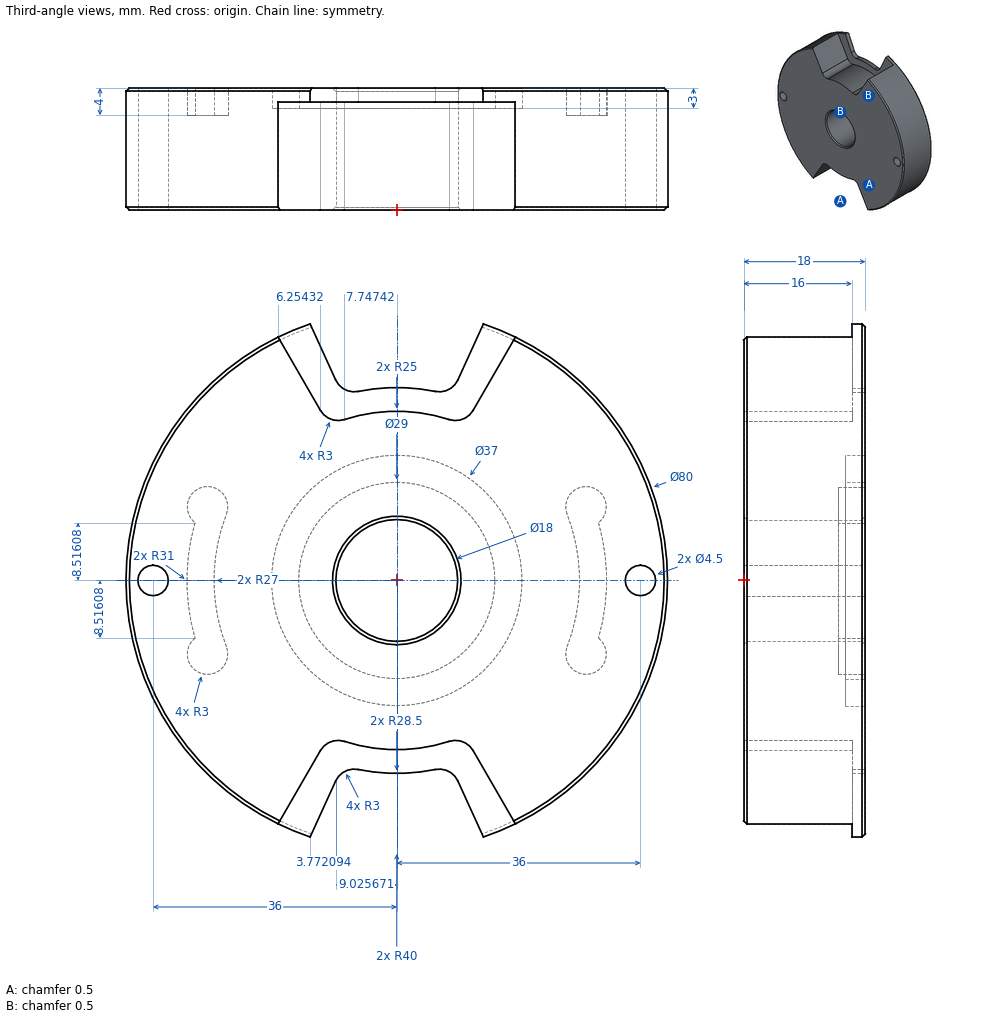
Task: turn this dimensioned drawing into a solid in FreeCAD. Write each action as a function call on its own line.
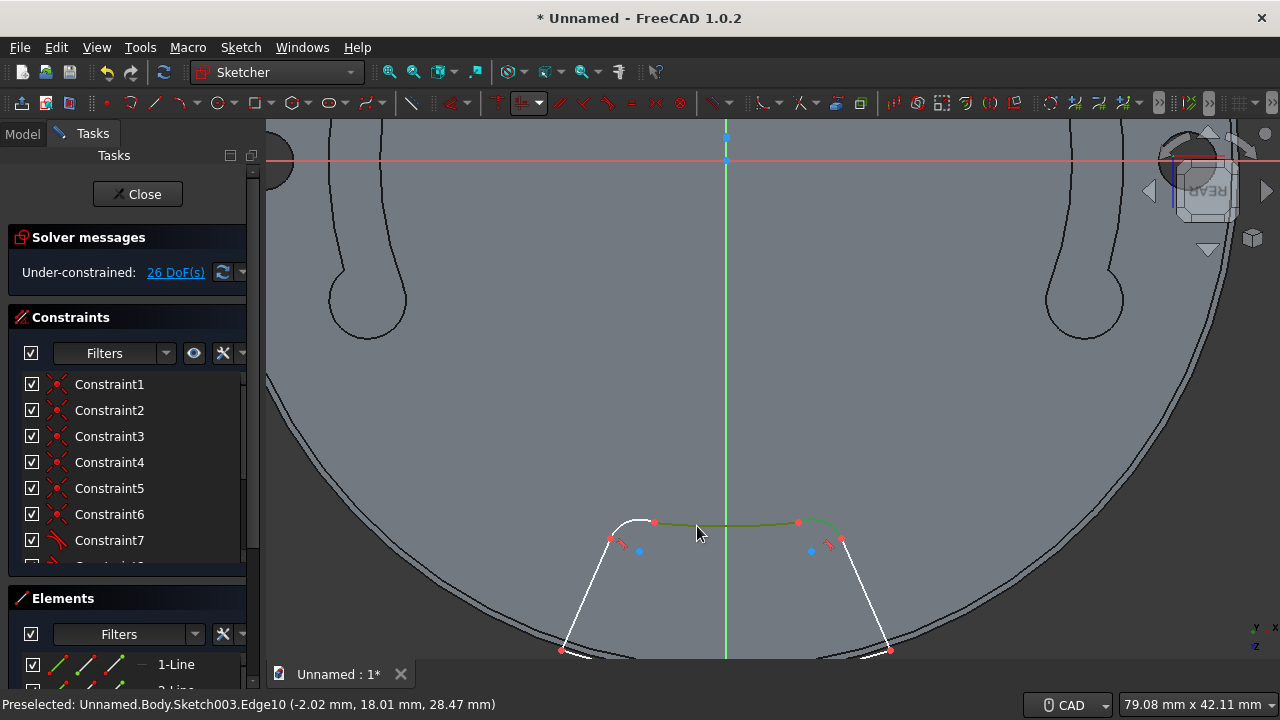
click(608, 104)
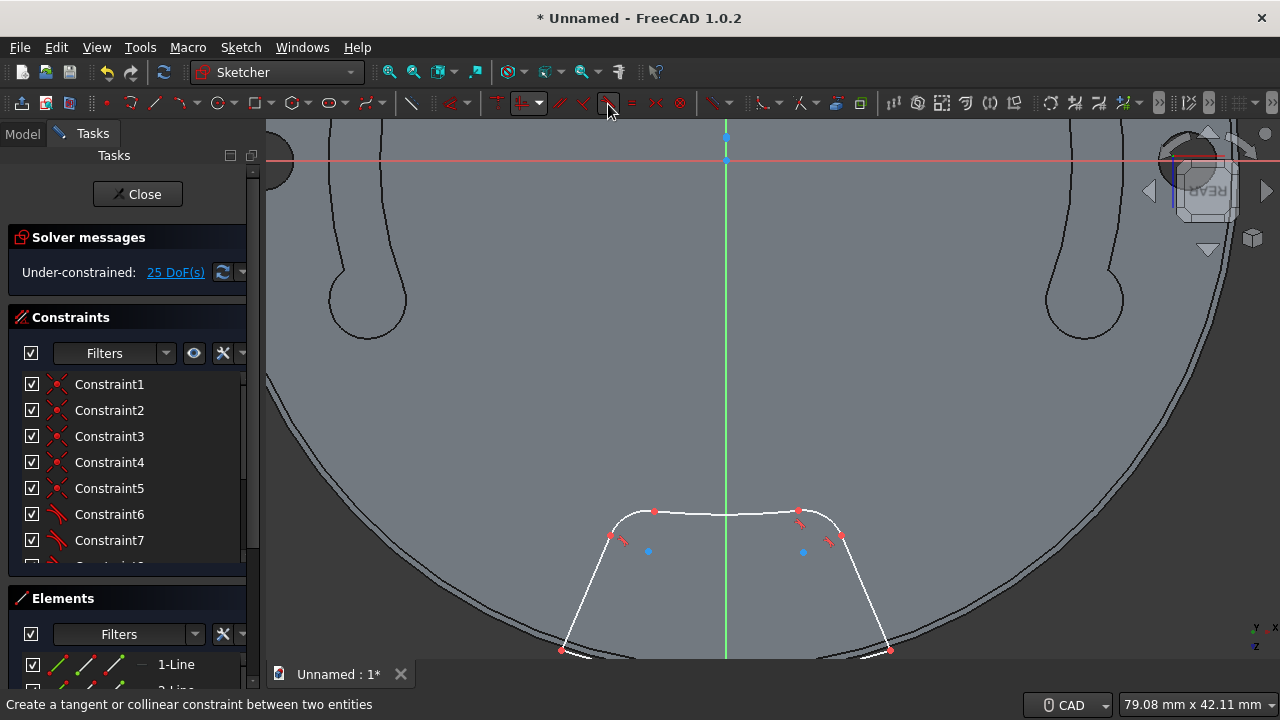
click(697, 514)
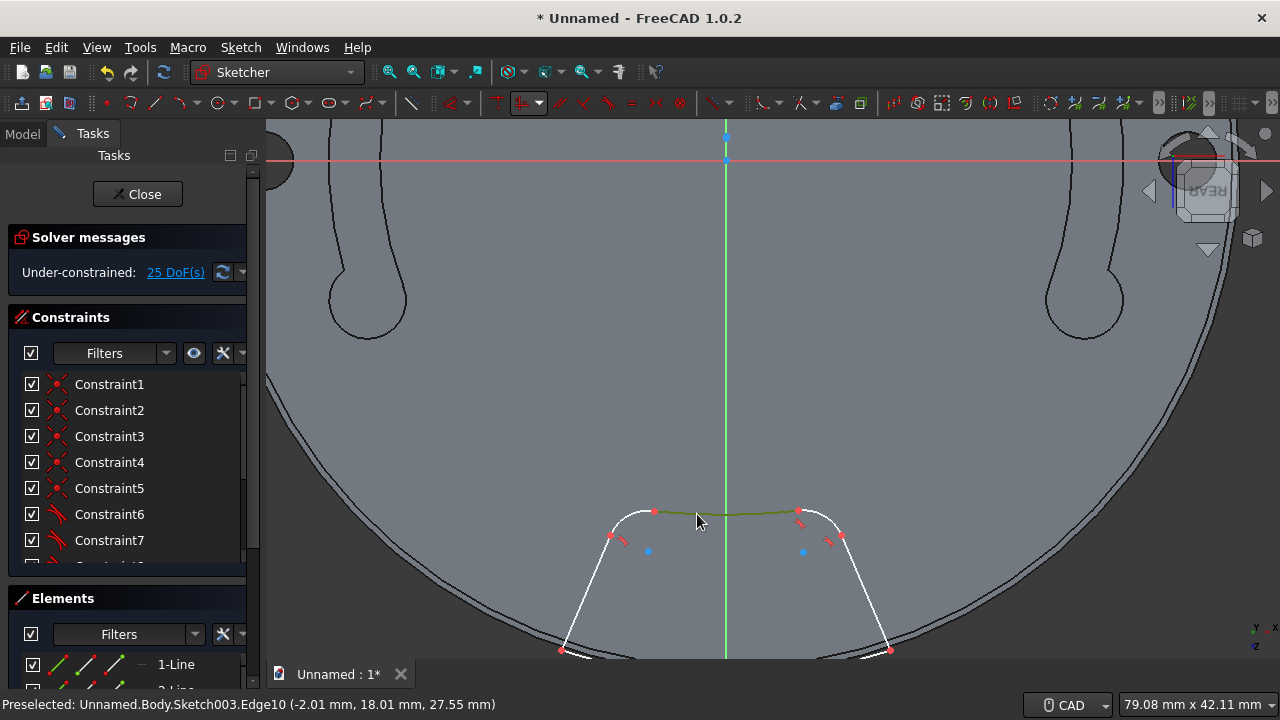
click(638, 512)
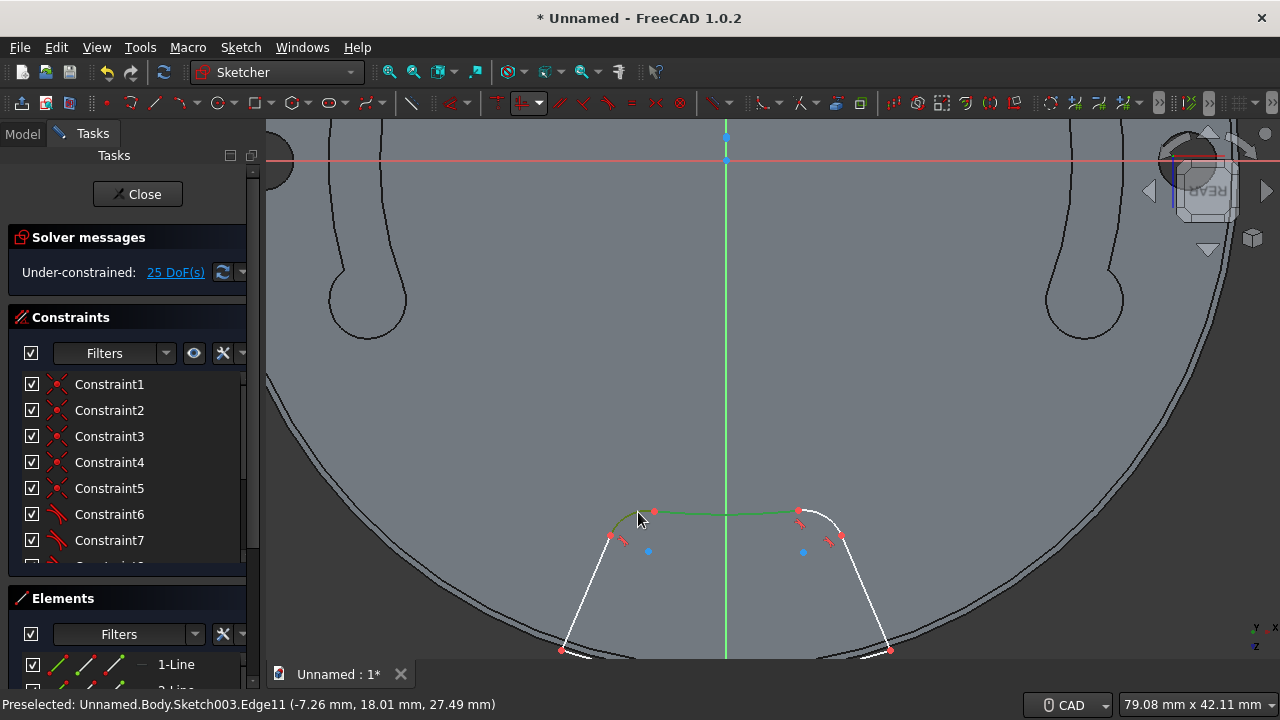
click(608, 104)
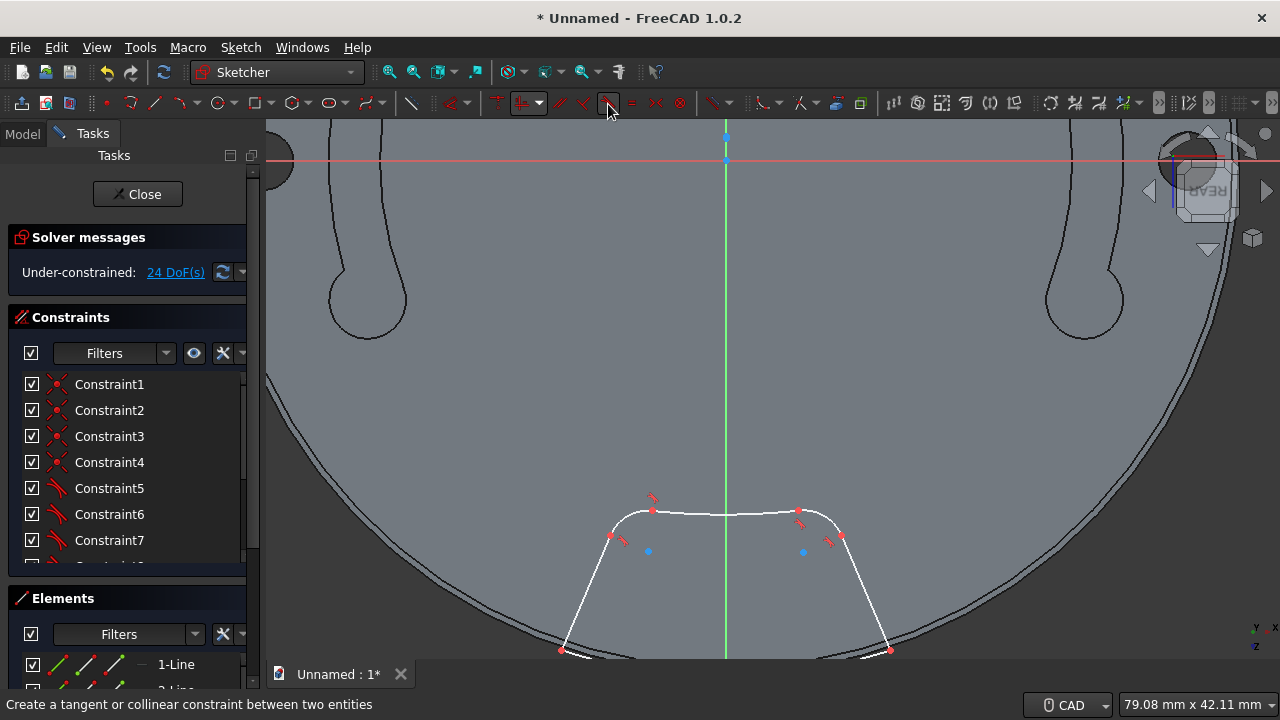
scroll(692, 522, down, 5)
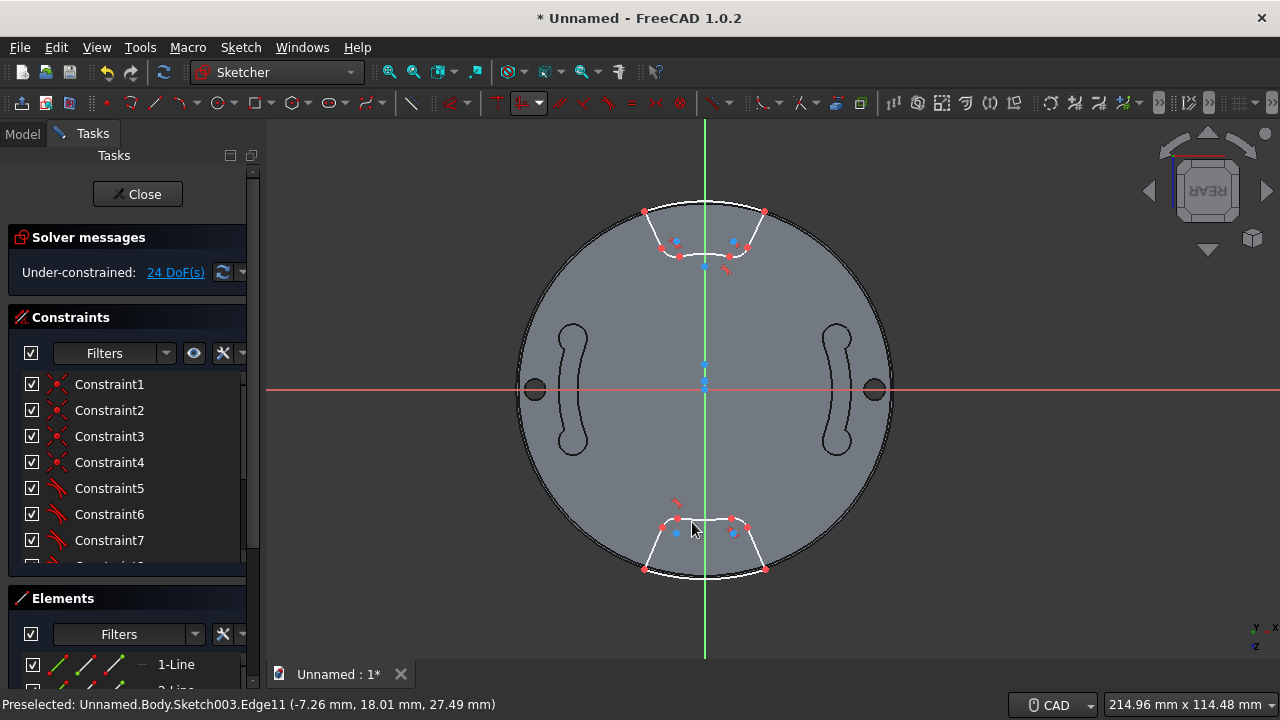
scroll(715, 254, up, 2)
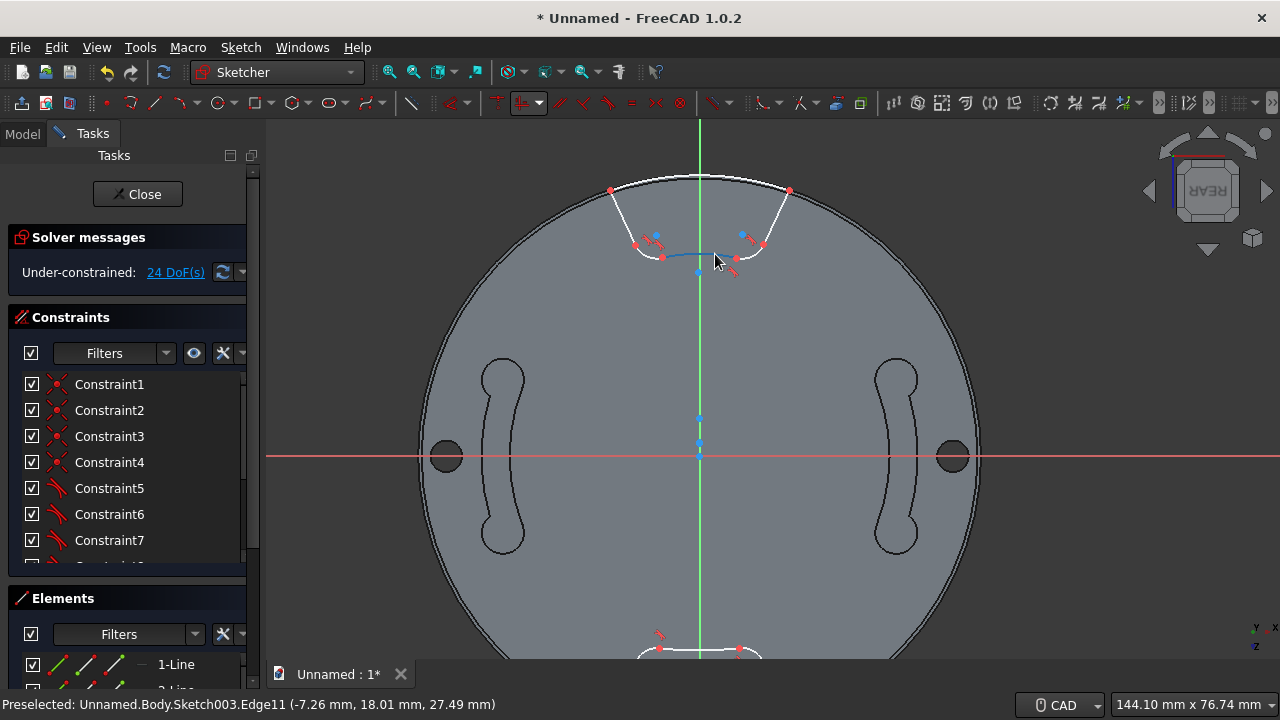
click(714, 254)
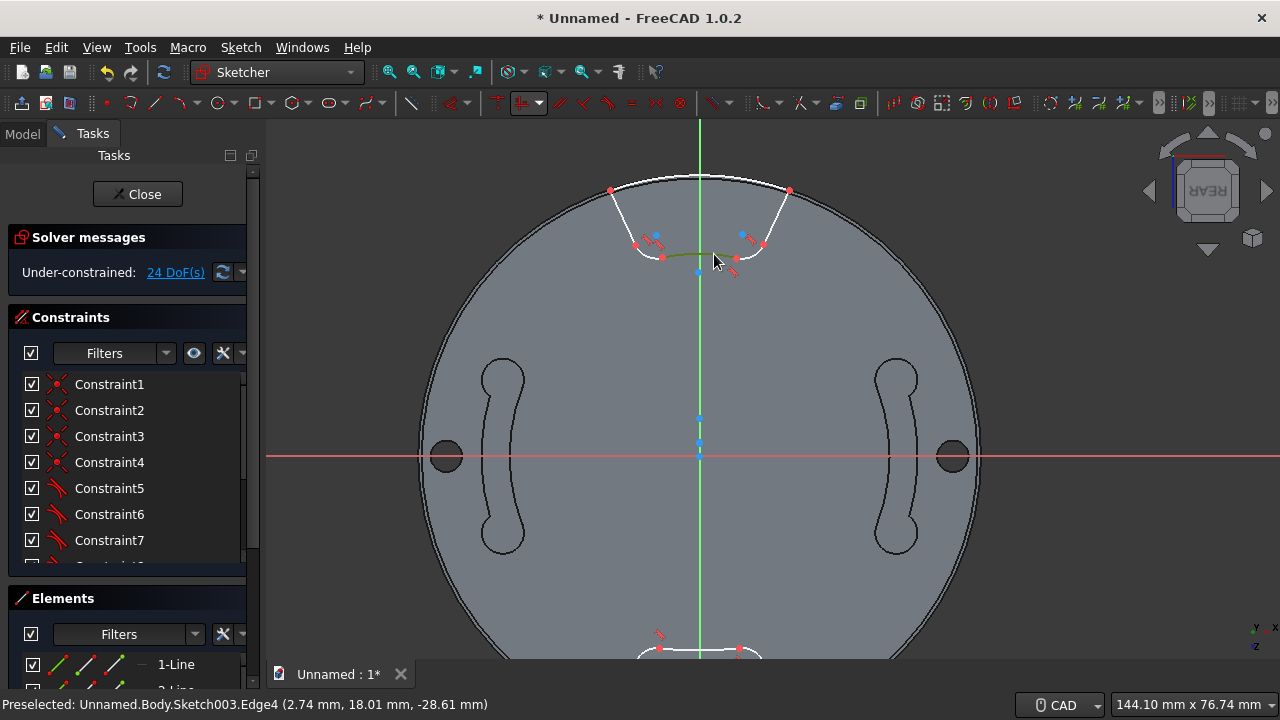
click(736, 178)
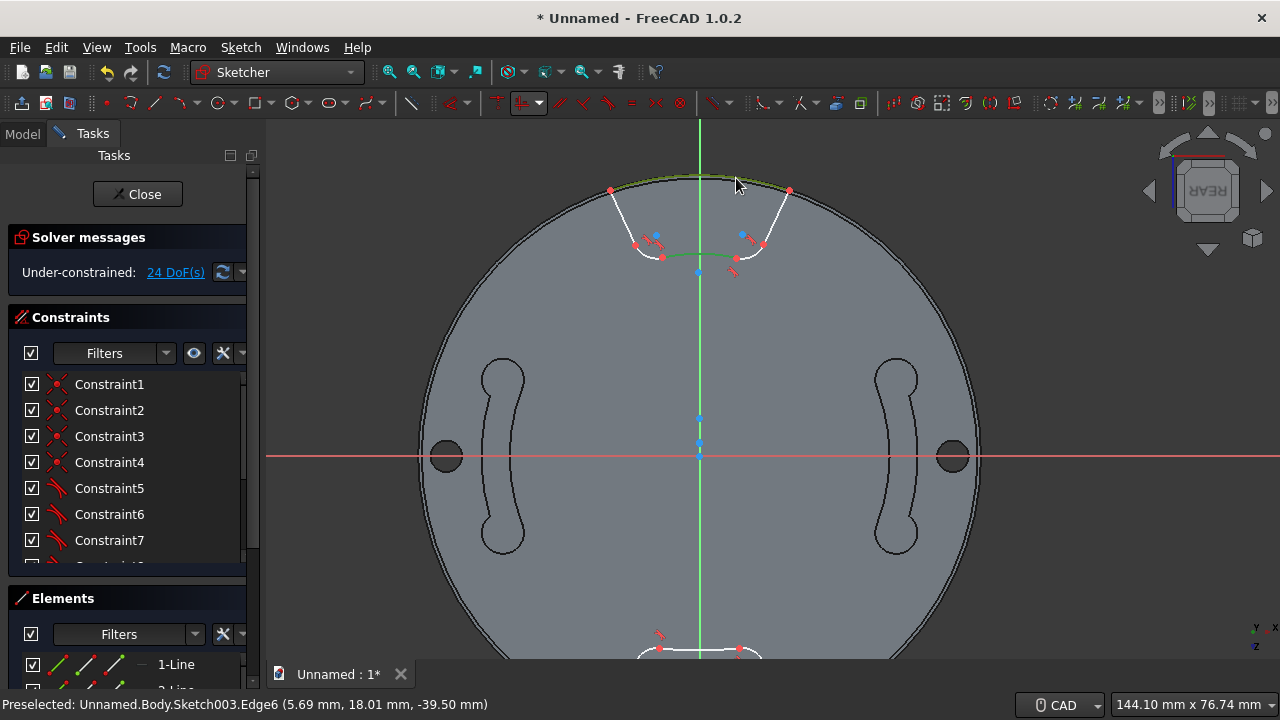
click(498, 104)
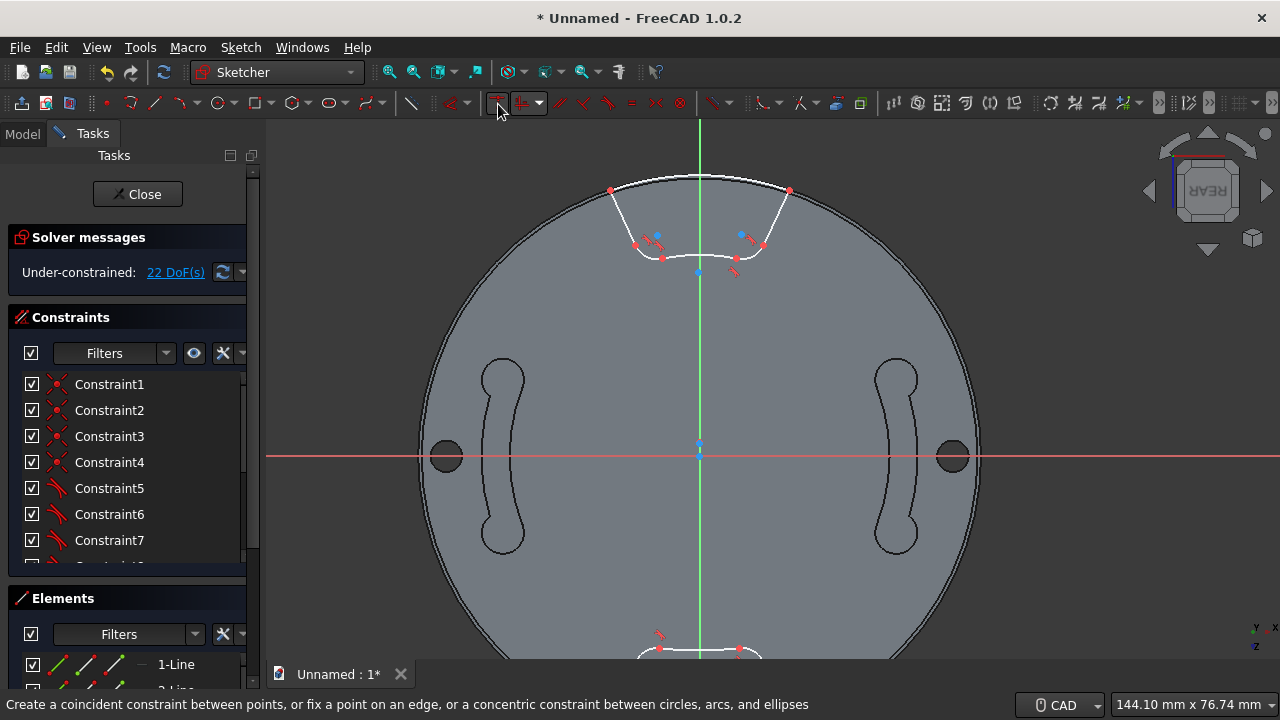
click(714, 256)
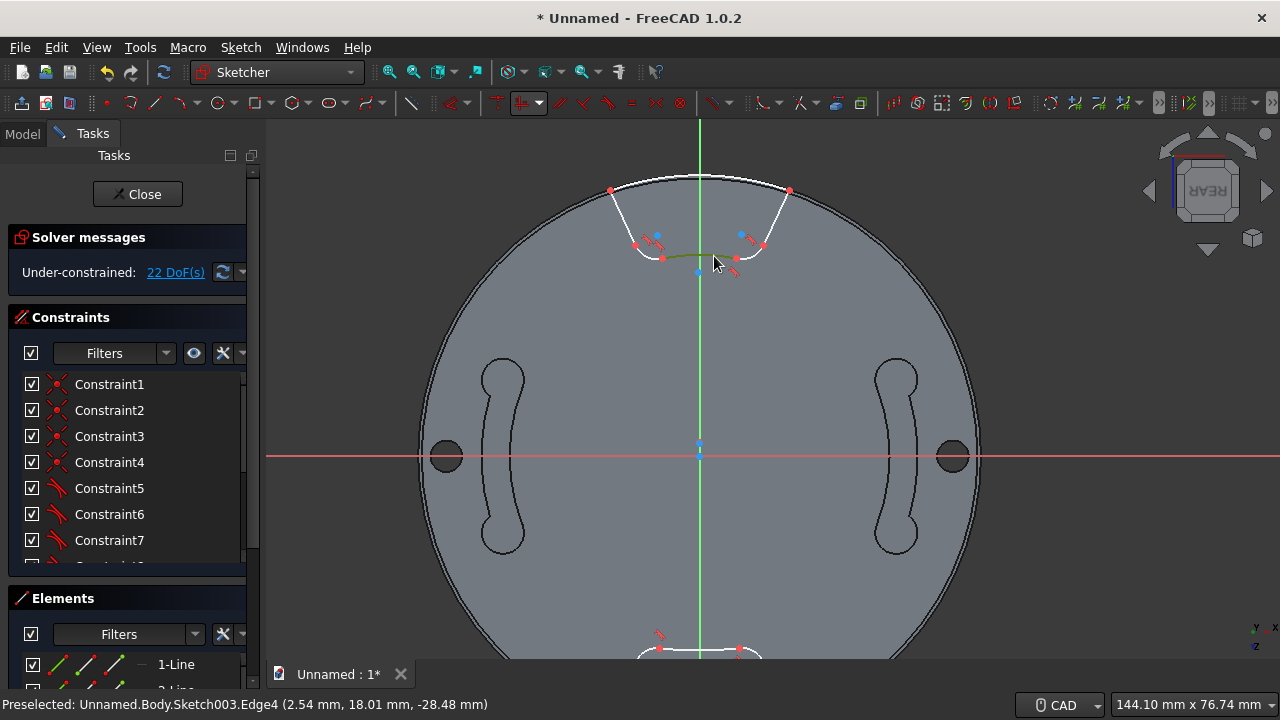
scroll(714, 252, down, 2)